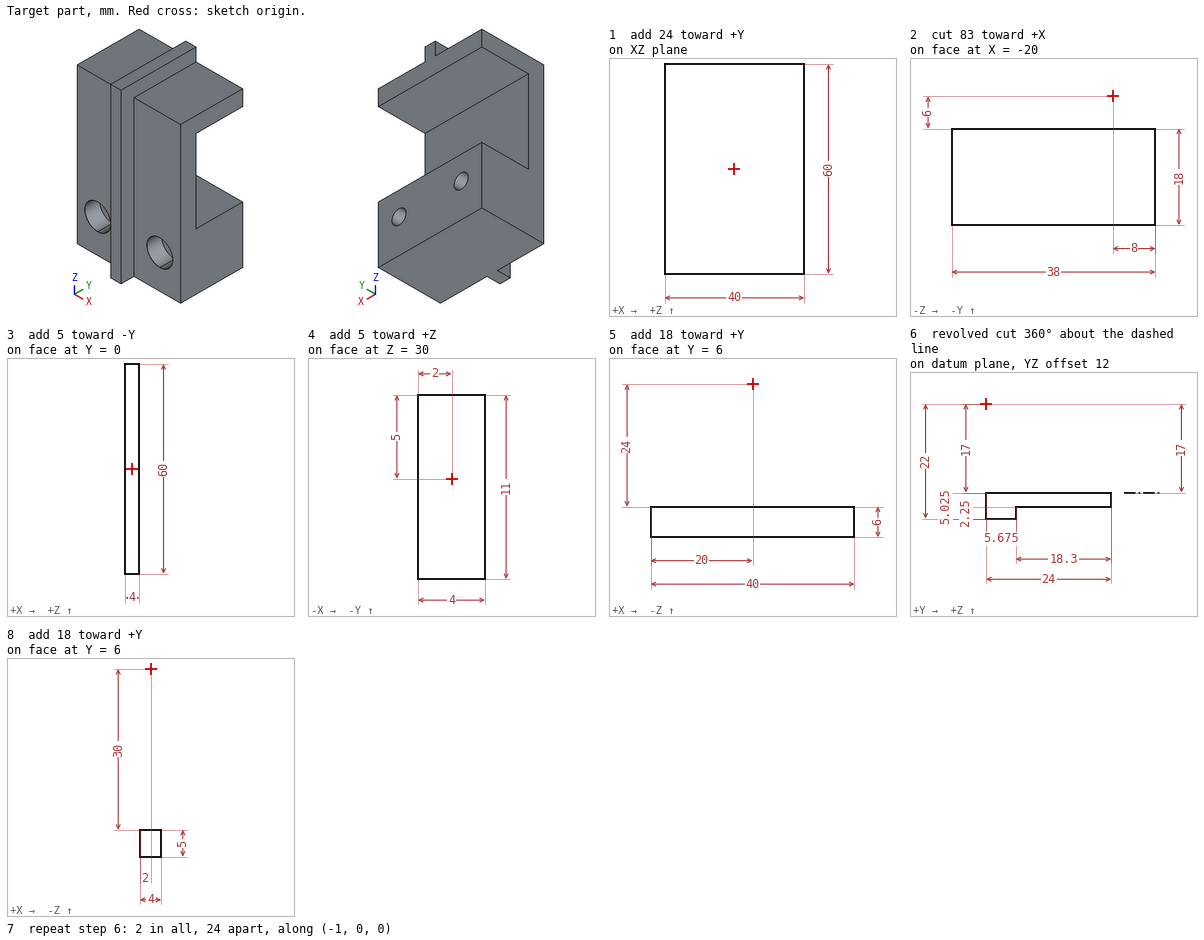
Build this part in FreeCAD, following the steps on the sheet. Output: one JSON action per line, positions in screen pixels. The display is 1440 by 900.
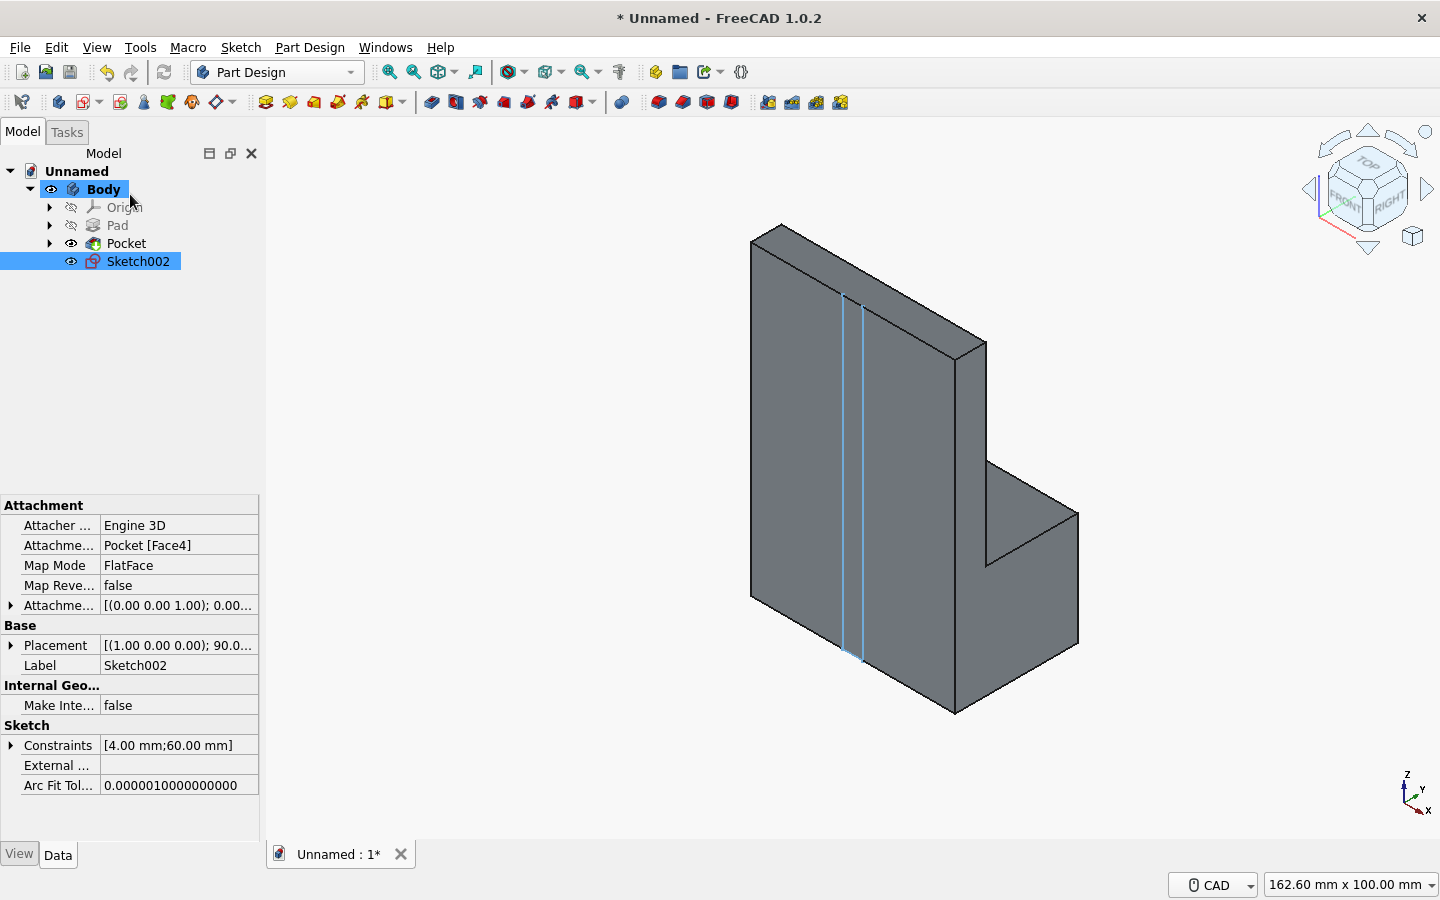
{"action": "left_click", "coordinate": [266, 102]}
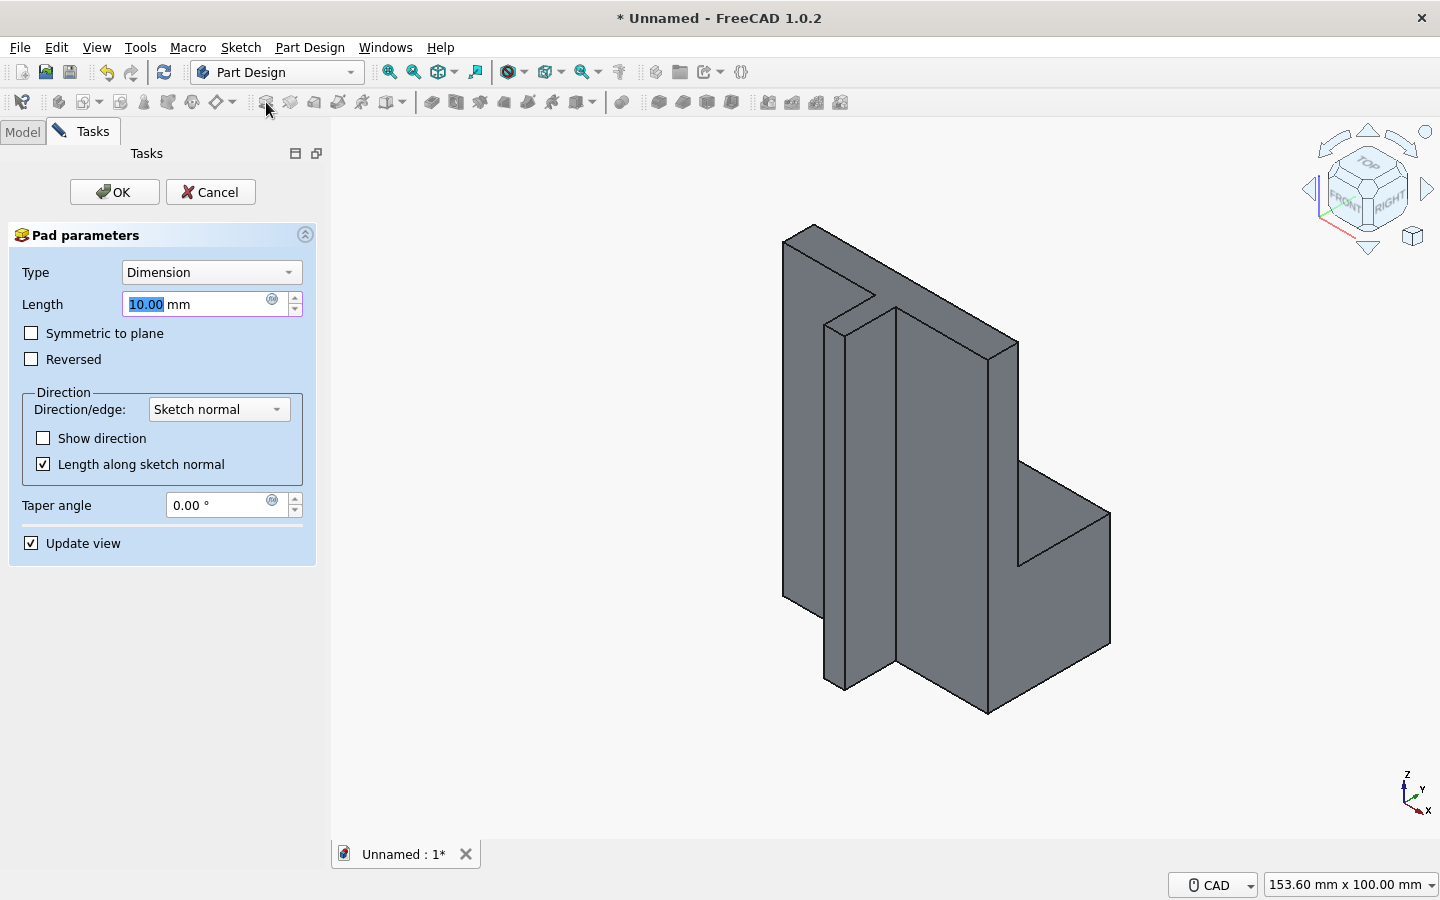
{"action": "type", "text": "5"}
{"action": "key", "text": "Tab"}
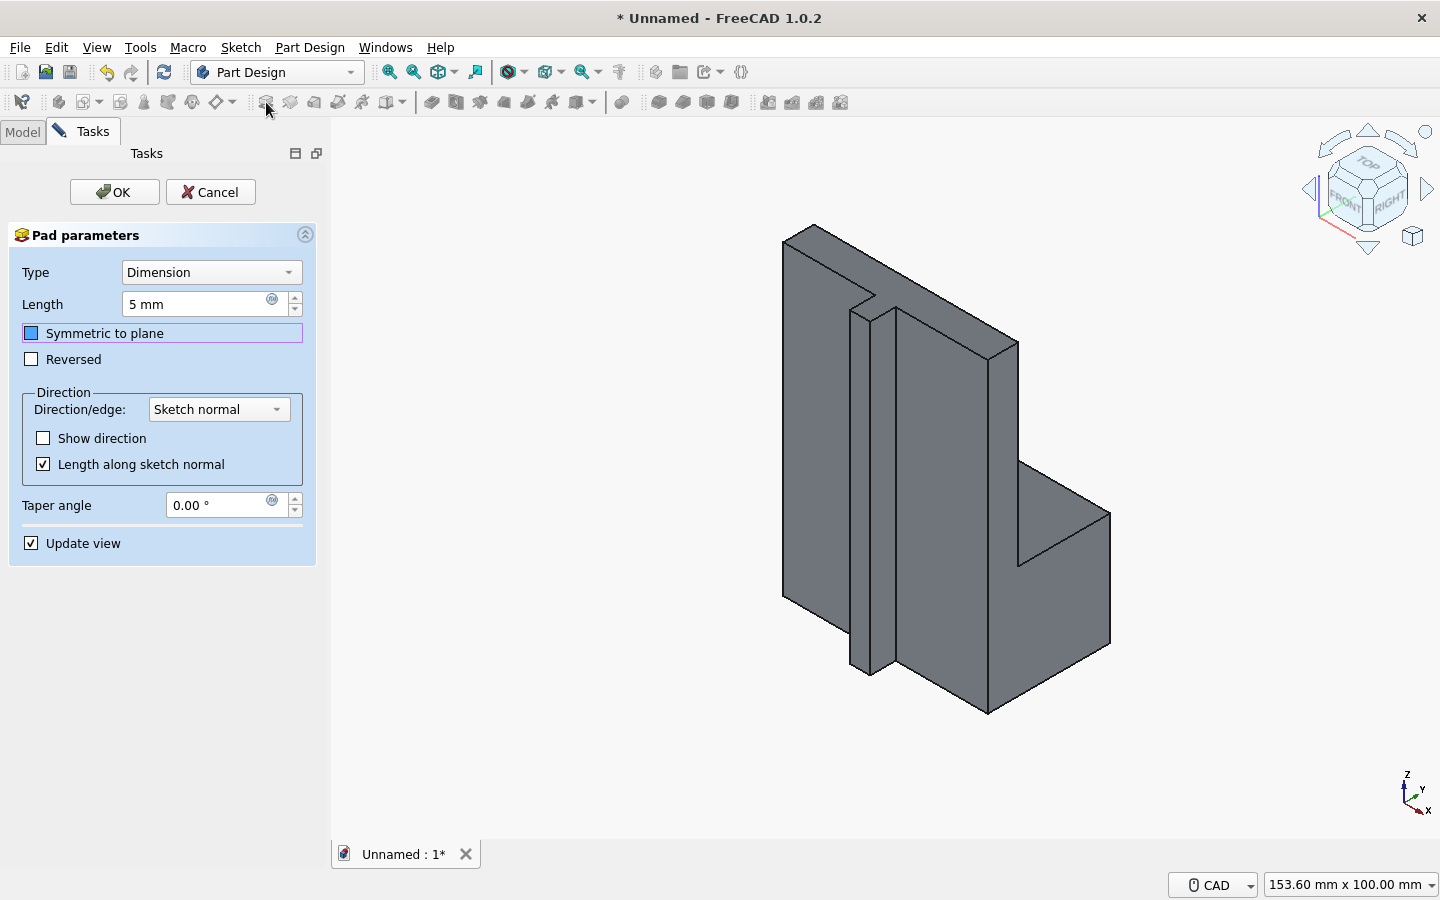
{"action": "left_click", "coordinate": [115, 192]}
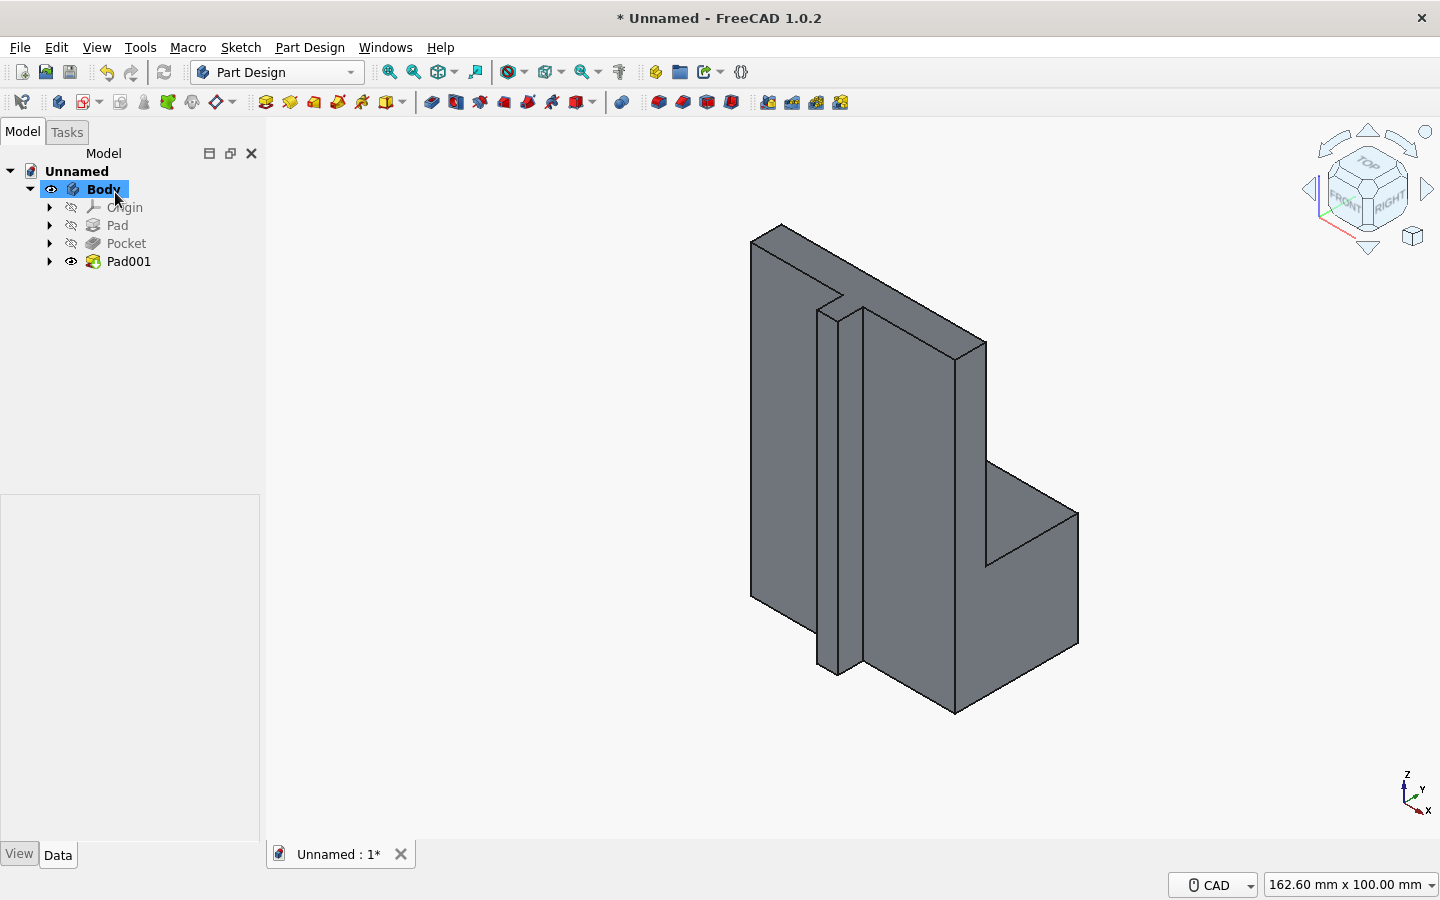
{"action": "left_click", "coordinate": [864, 294]}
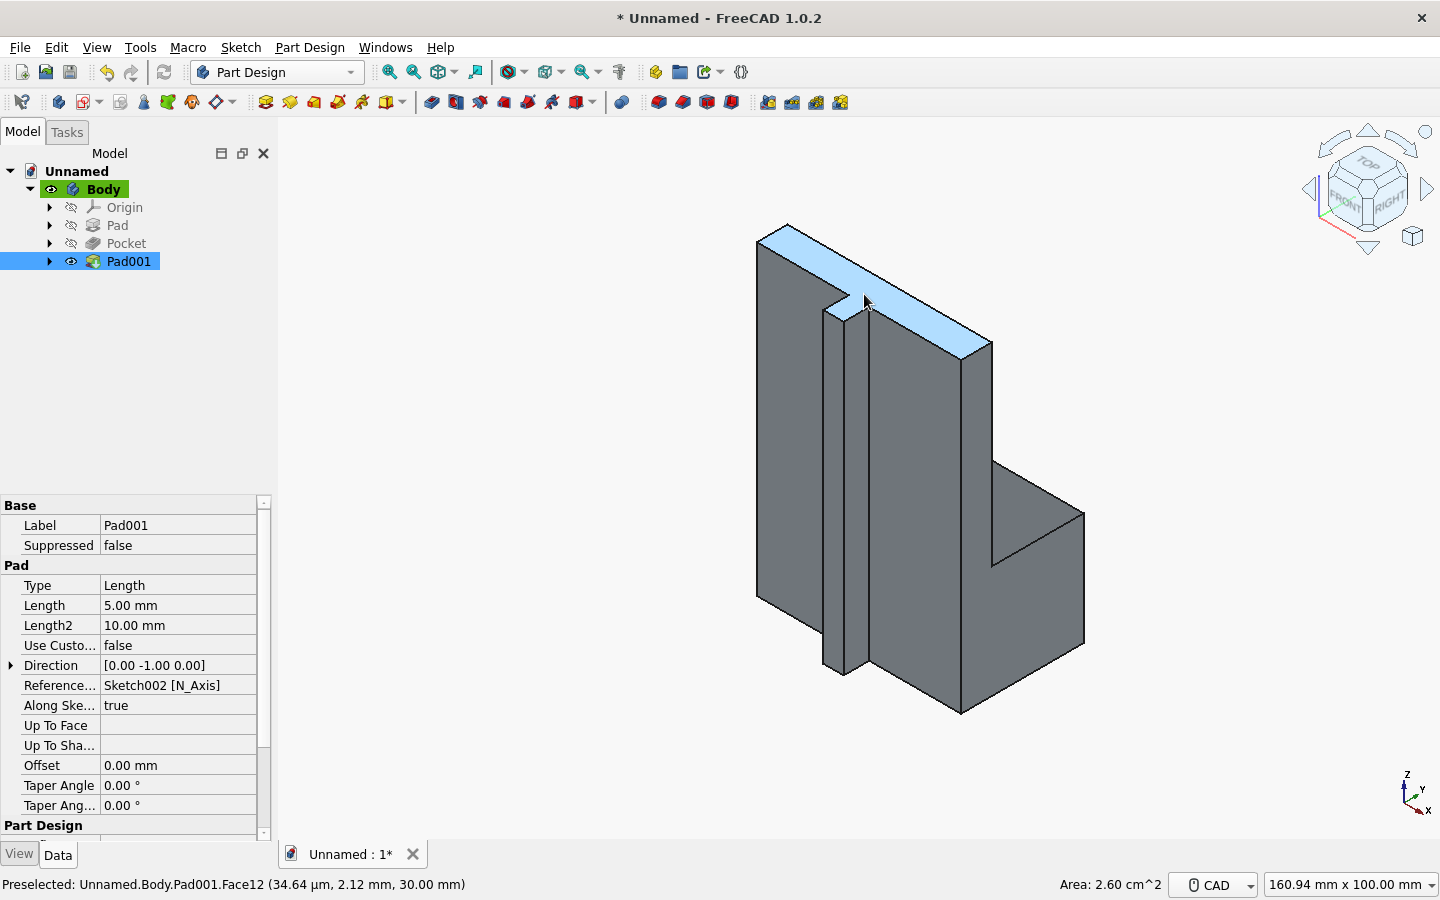
{"action": "left_click", "coordinate": [84, 102]}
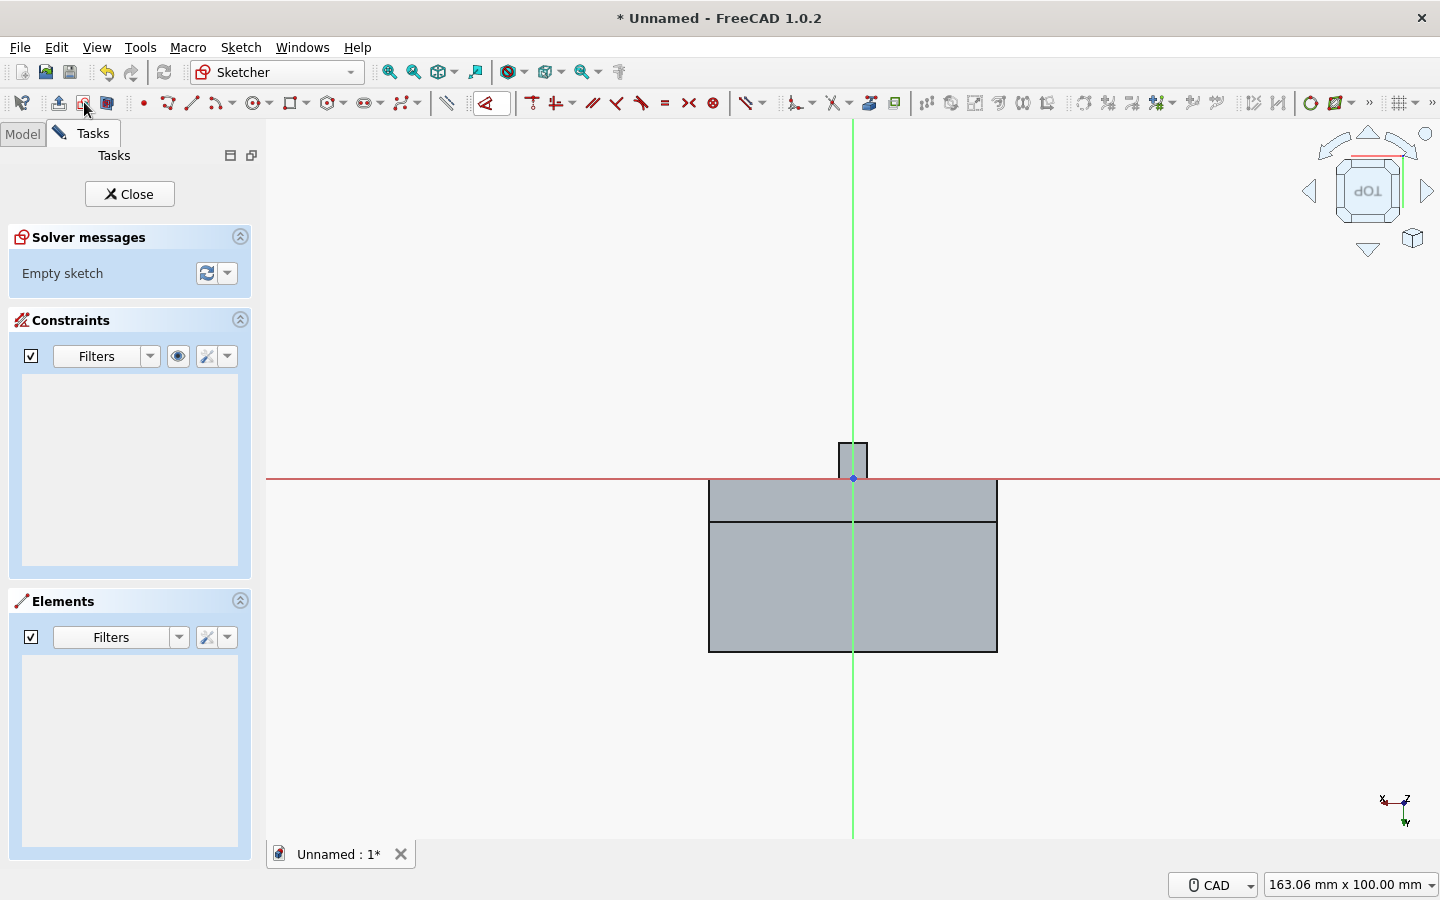
{"action": "scroll", "coordinate": [867, 483], "scroll_direction": "up", "scroll_amount": 9}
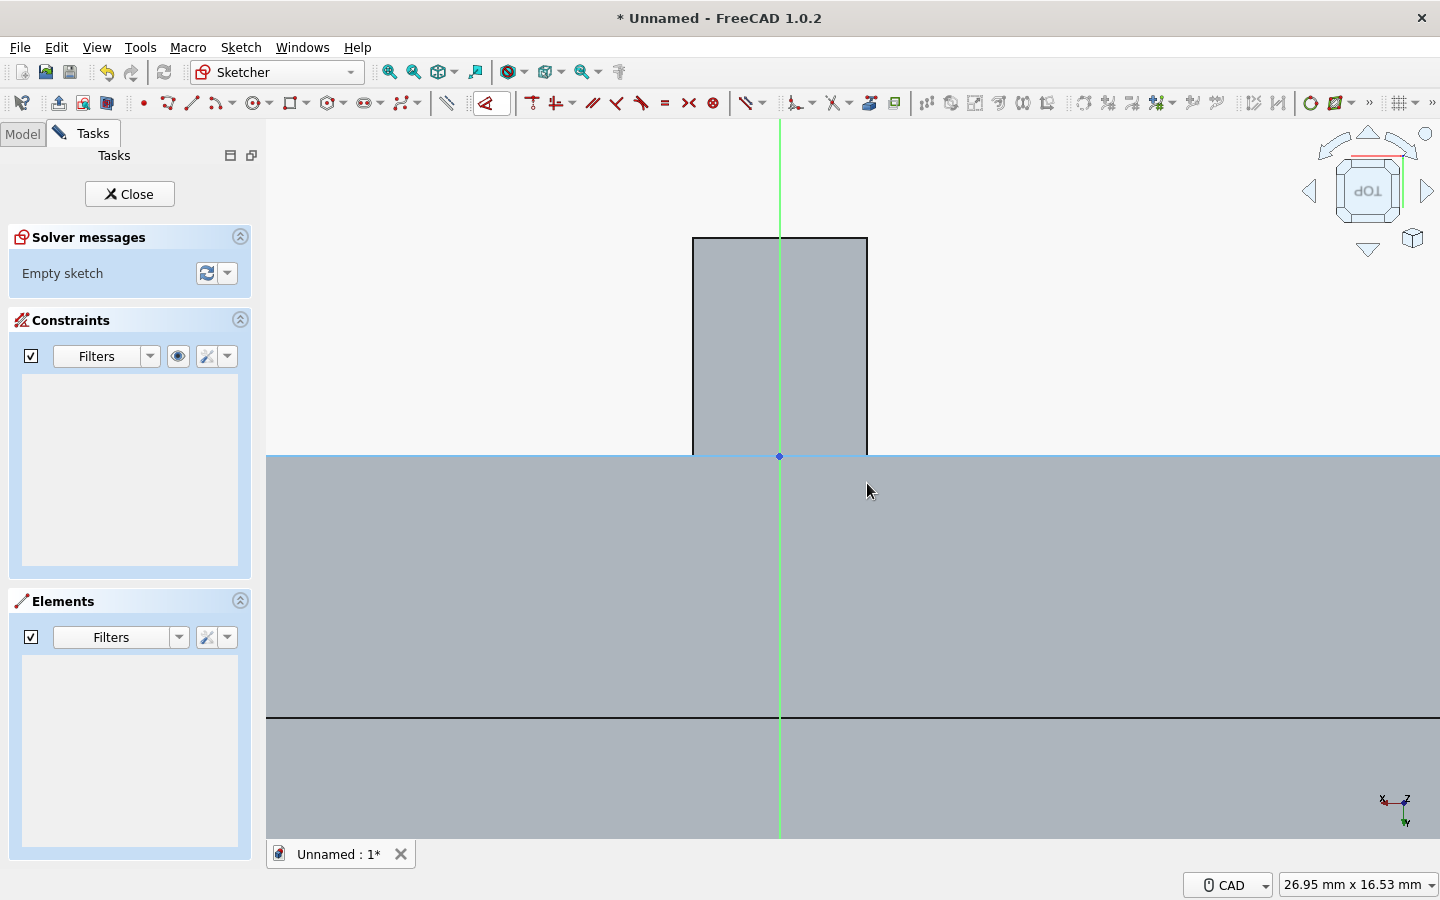
{"action": "key", "text": "g r"}